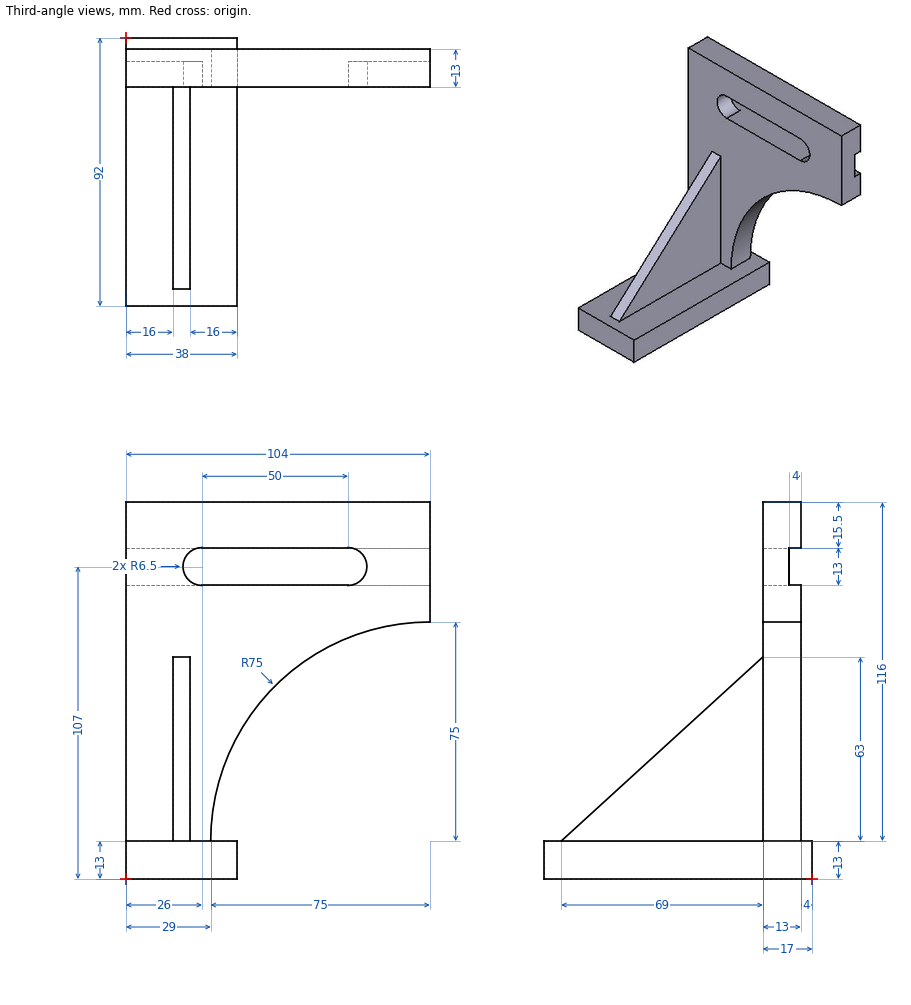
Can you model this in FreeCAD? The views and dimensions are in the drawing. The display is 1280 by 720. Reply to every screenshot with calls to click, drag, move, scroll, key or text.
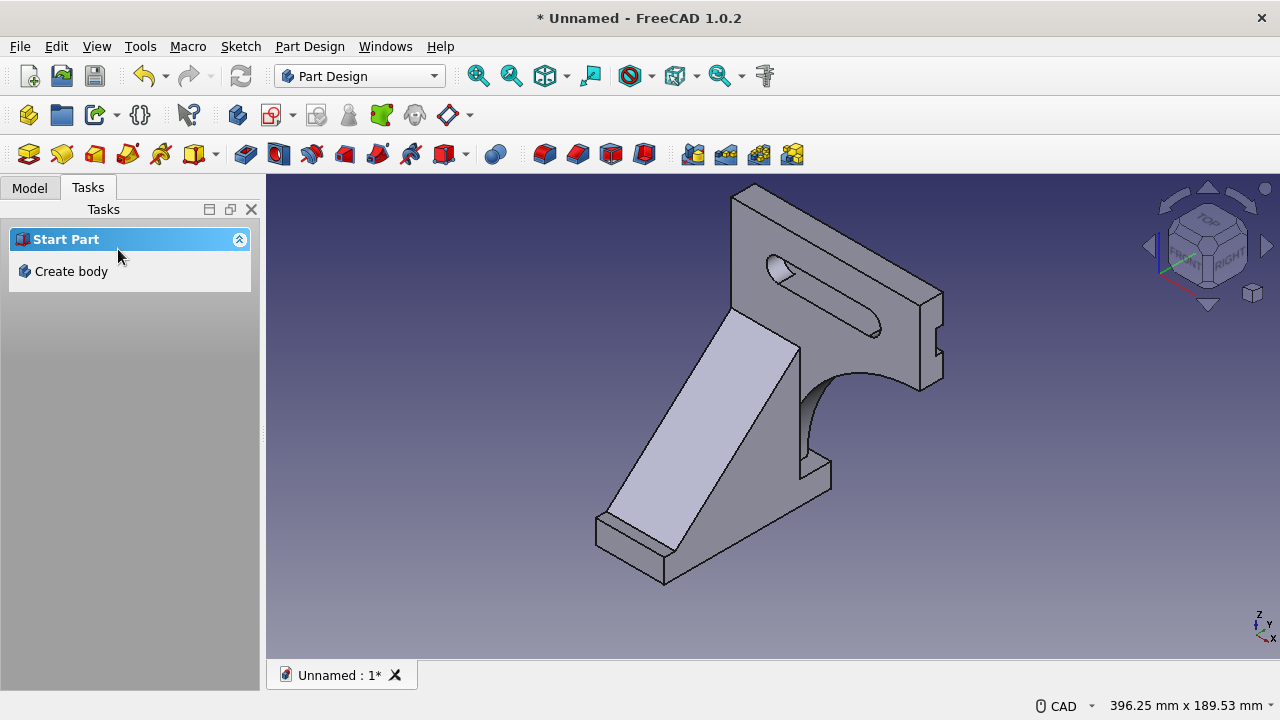
click(748, 479)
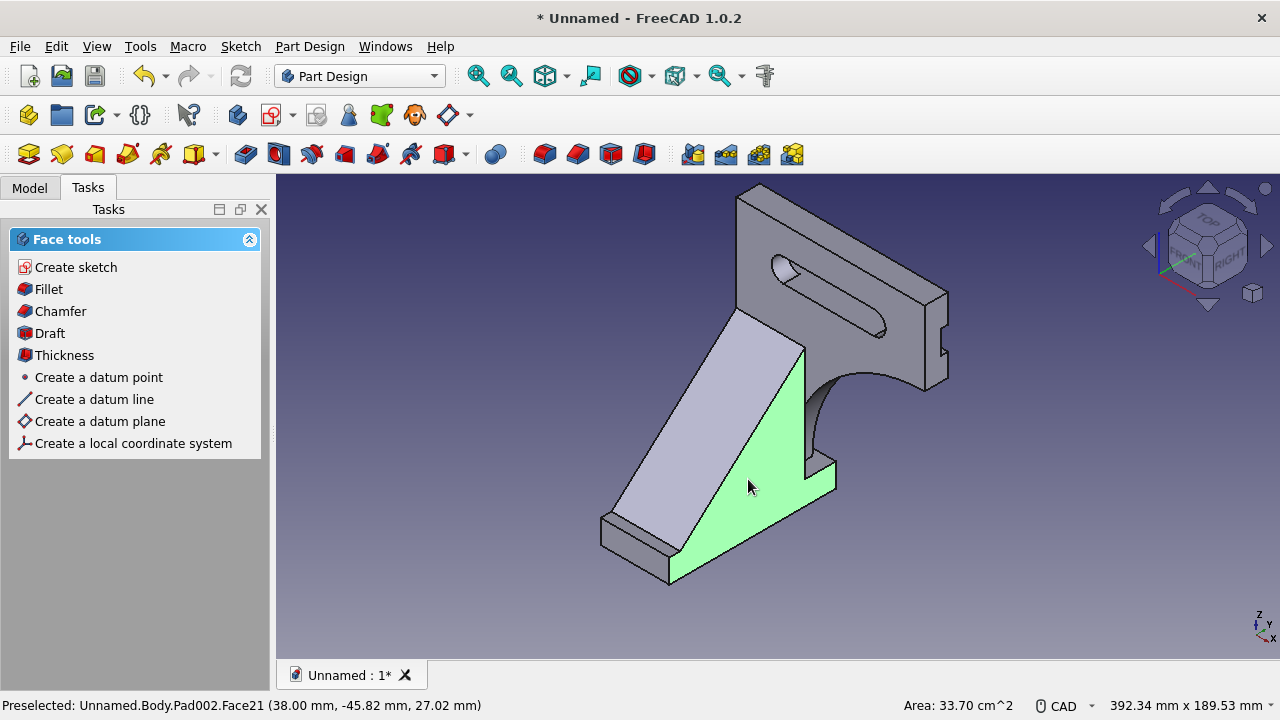
click(270, 116)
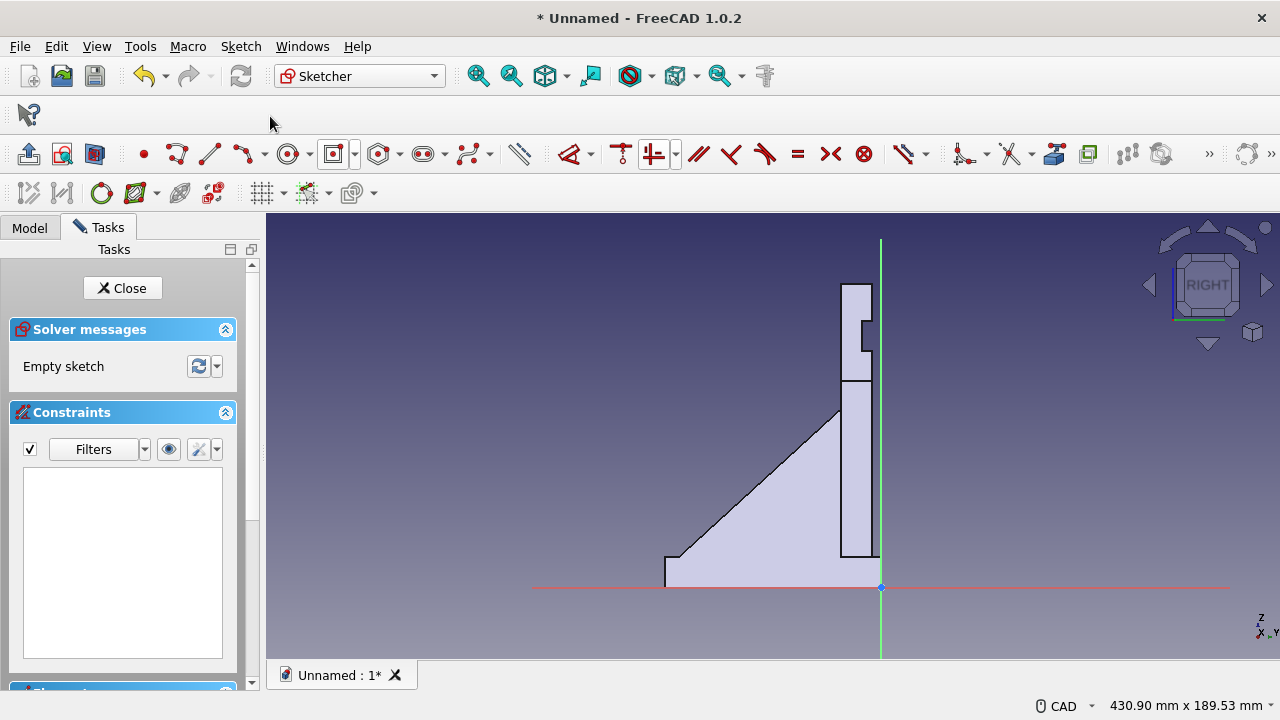
scroll(934, 625, up, 2)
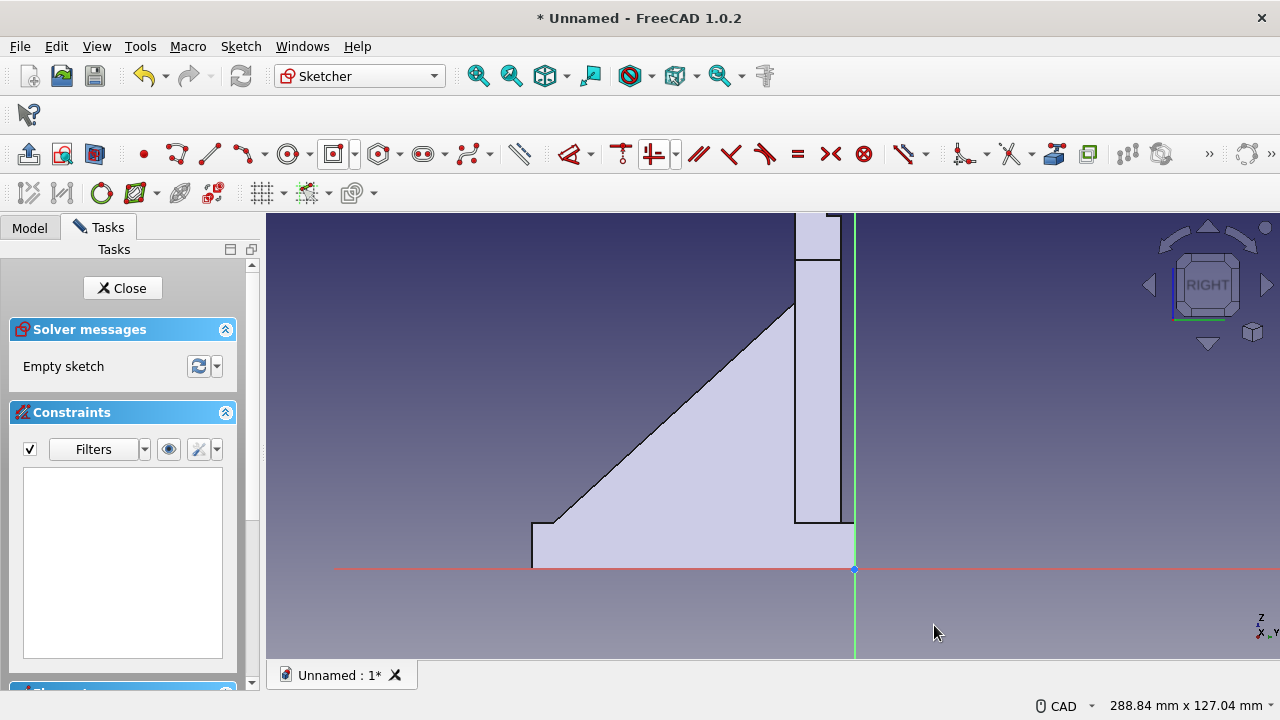
click(177, 154)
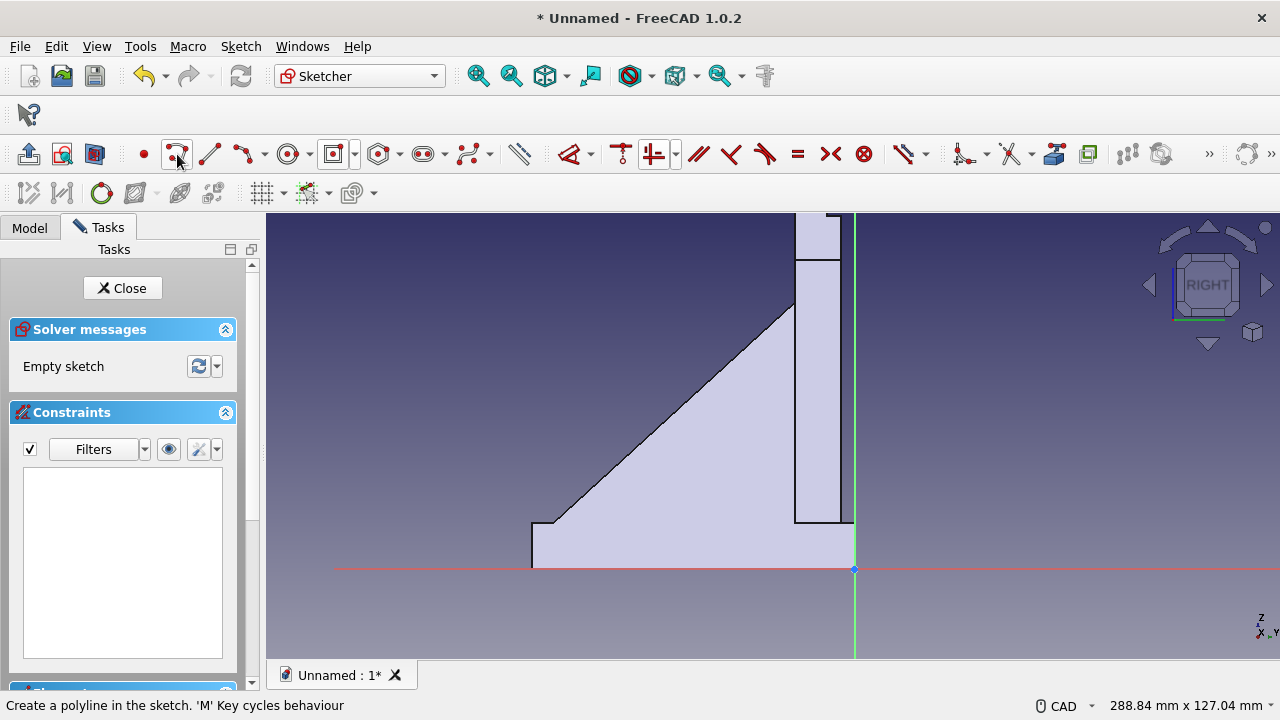
click(795, 523)
click(795, 302)
click(553, 523)
click(795, 524)
key(Escape)
key(Escape)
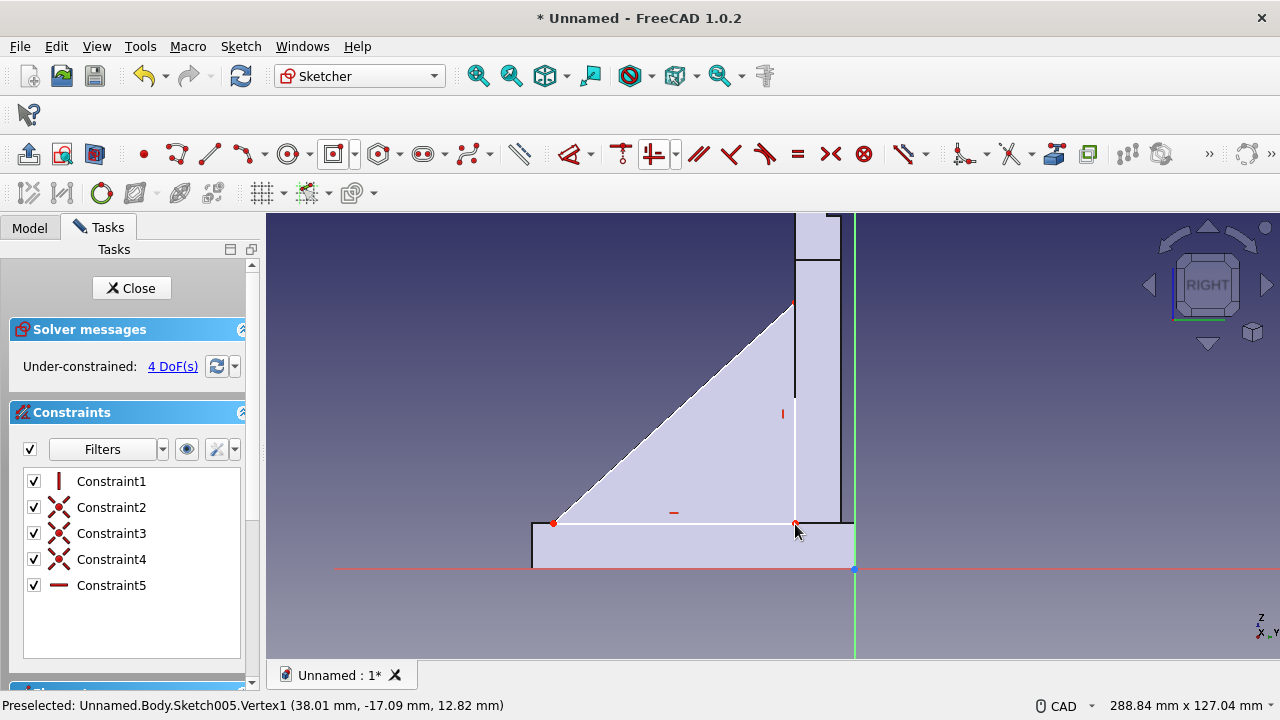
click(568, 154)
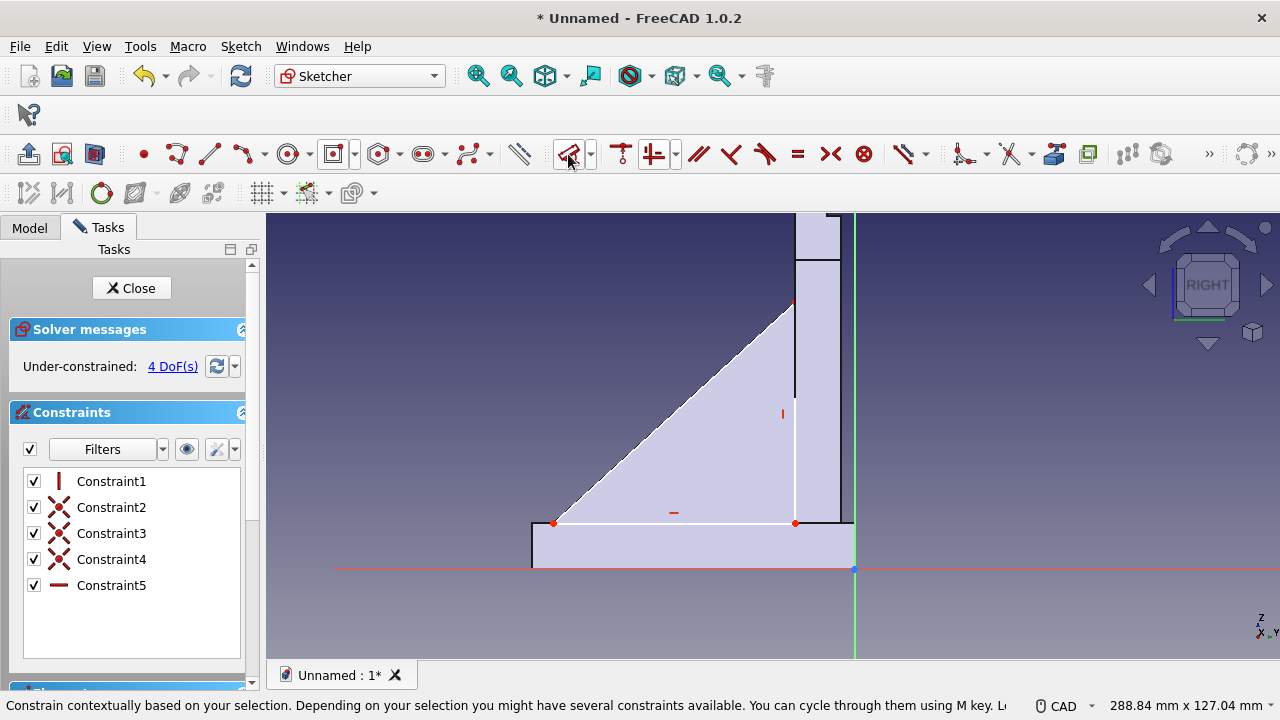
click(795, 458)
click(829, 414)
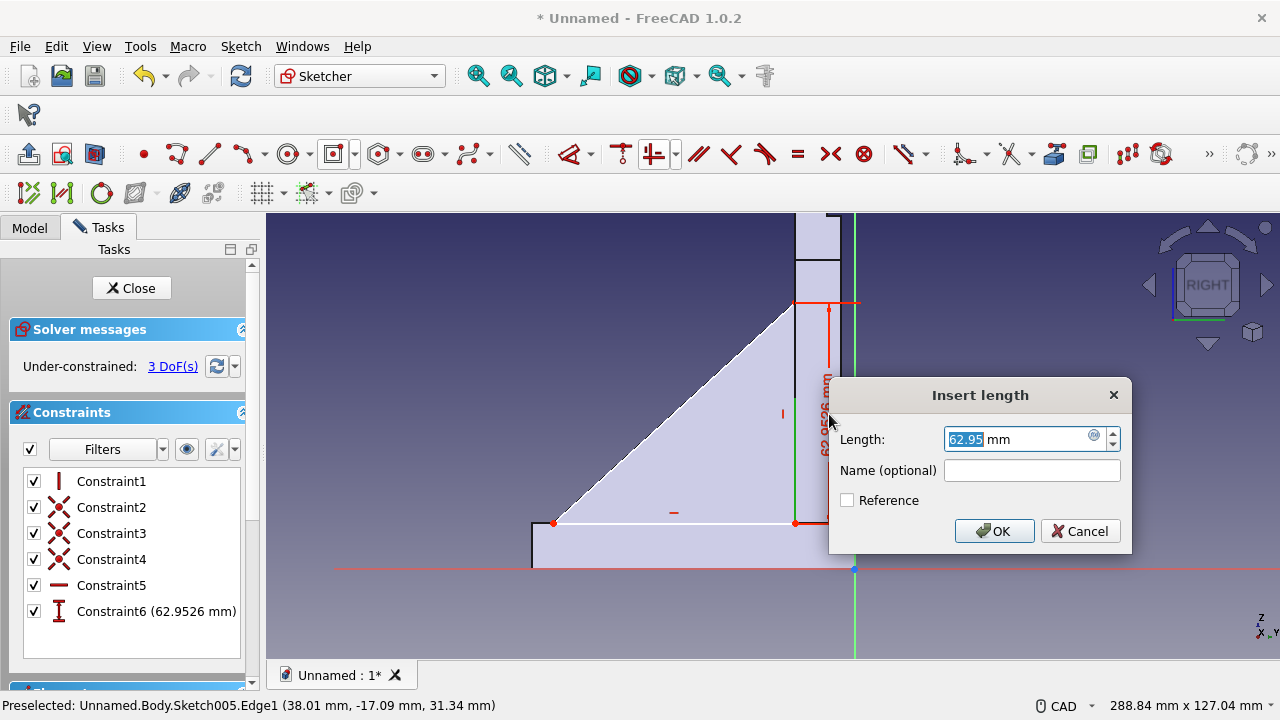
text(63)
key(Return)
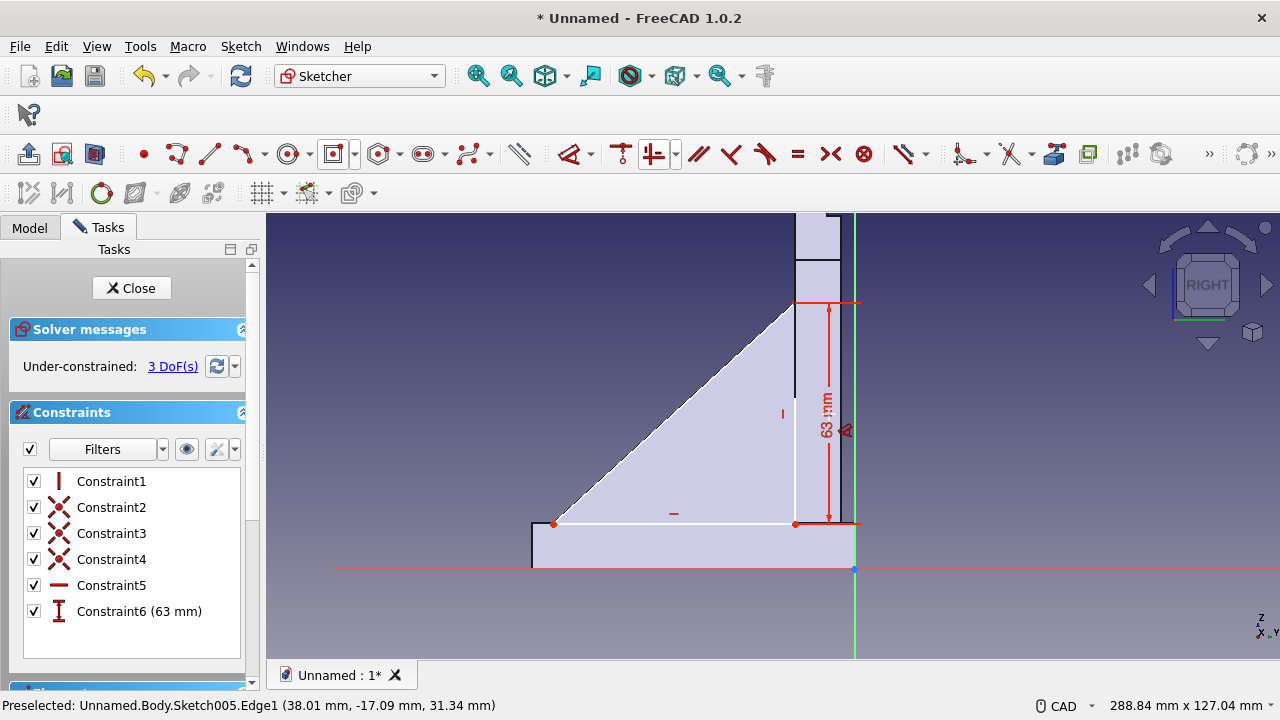
click(626, 524)
click(674, 490)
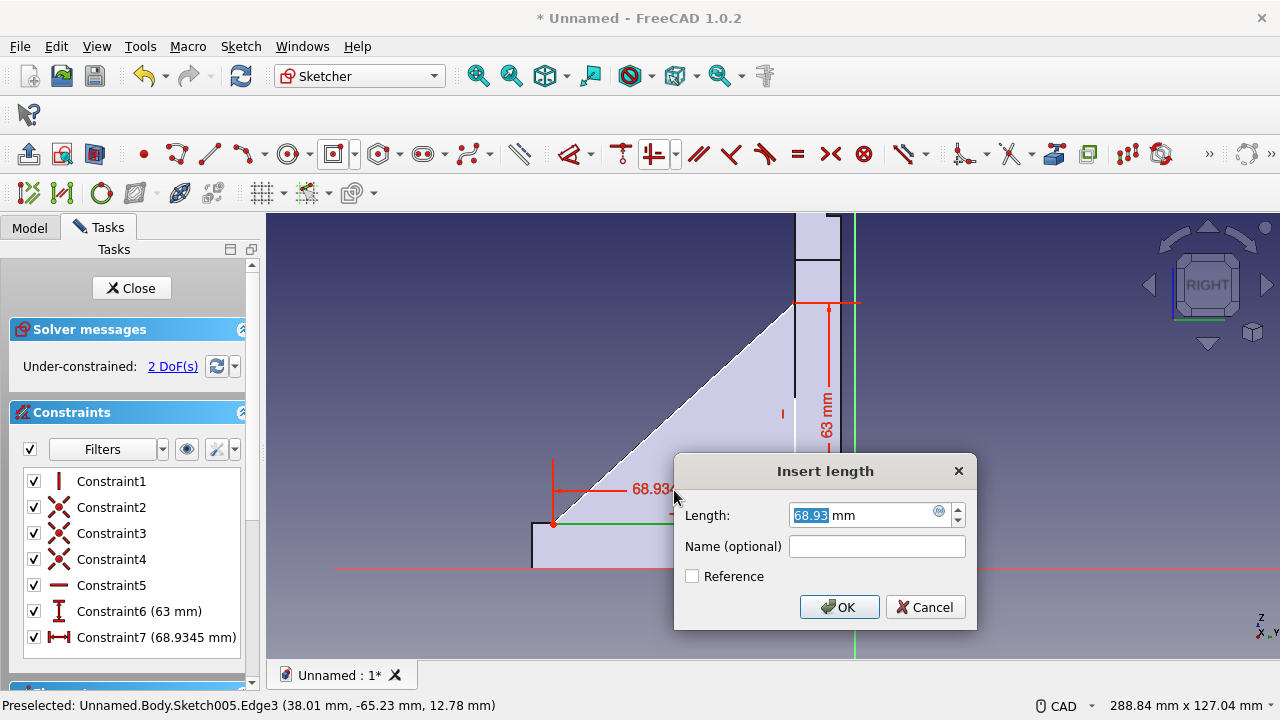
text(69)
key(Return)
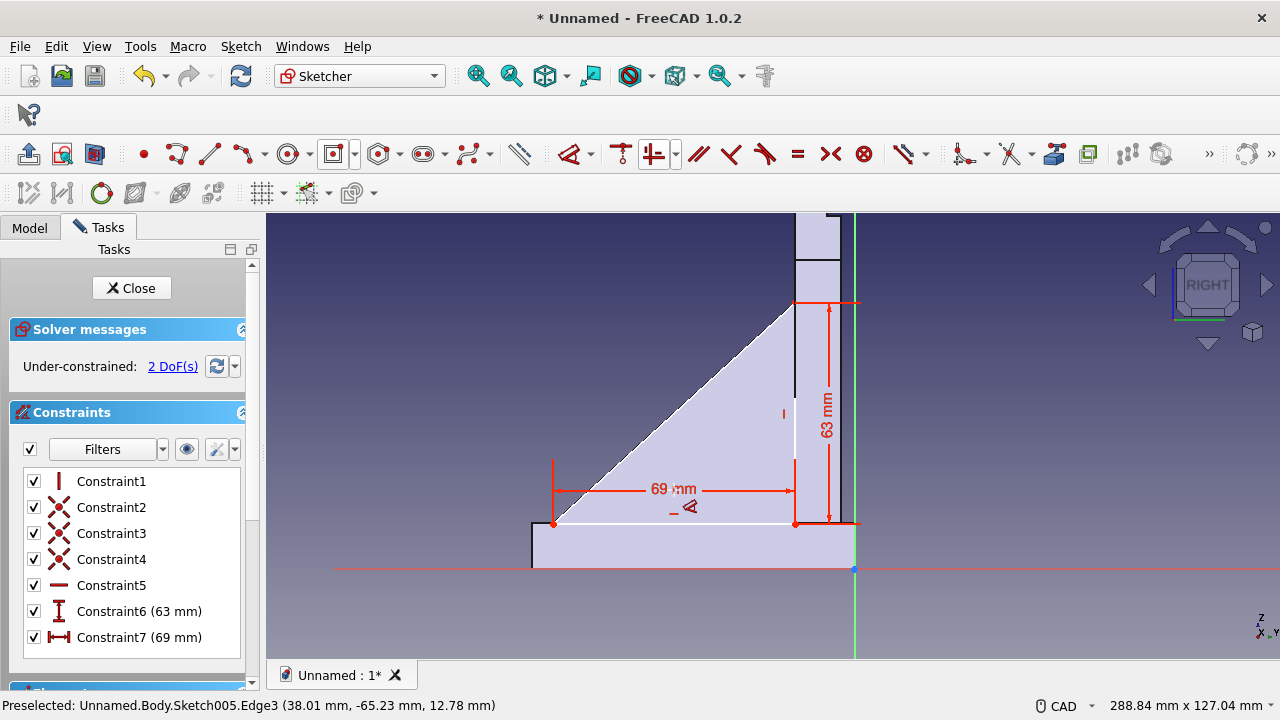
click(795, 524)
click(825, 603)